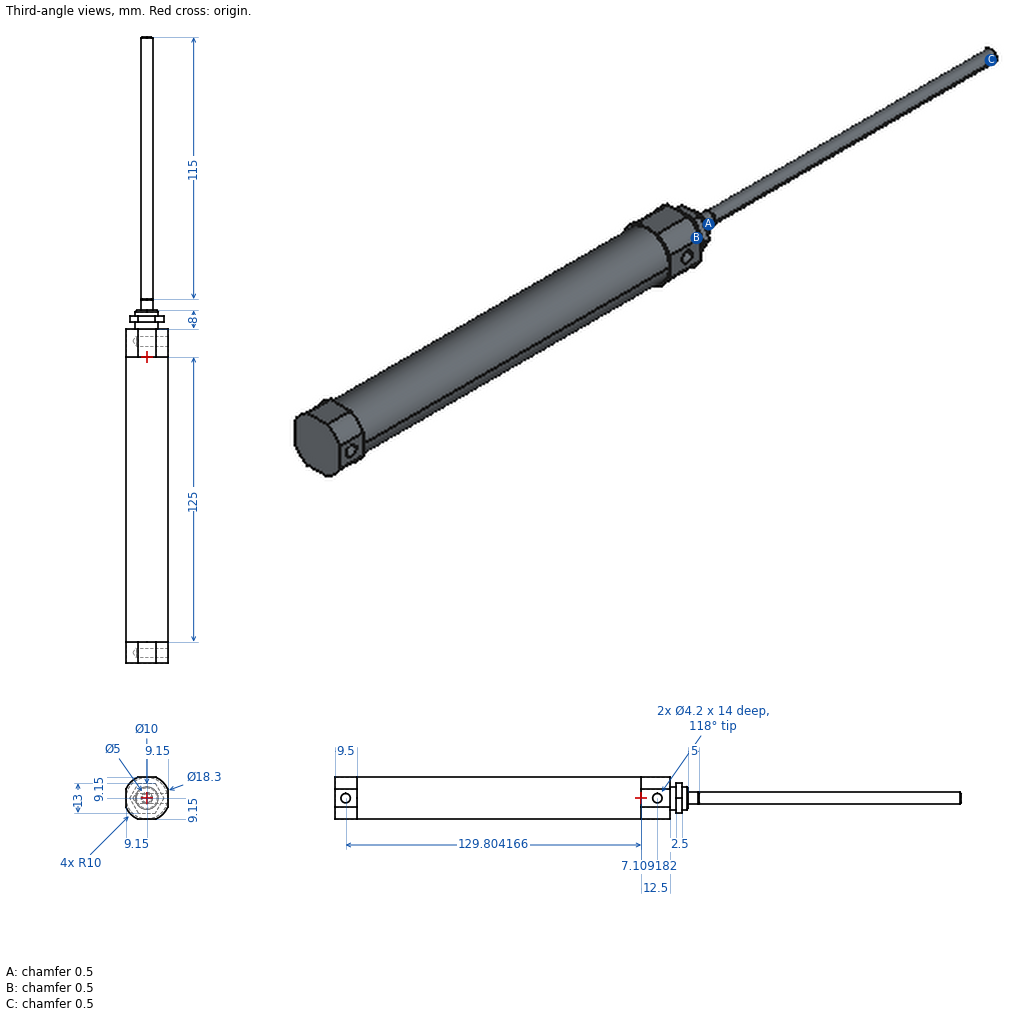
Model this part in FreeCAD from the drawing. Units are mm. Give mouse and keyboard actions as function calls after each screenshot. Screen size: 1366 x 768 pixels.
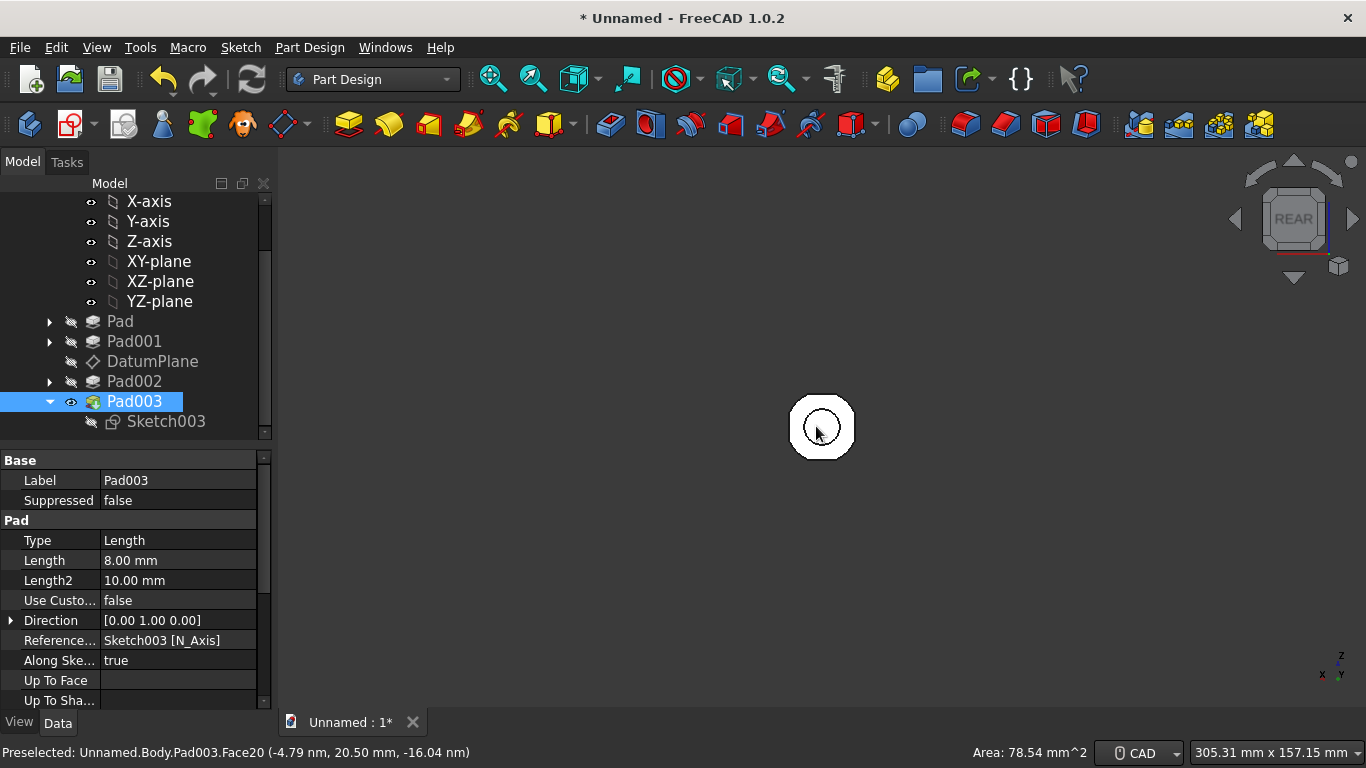
click(70, 124)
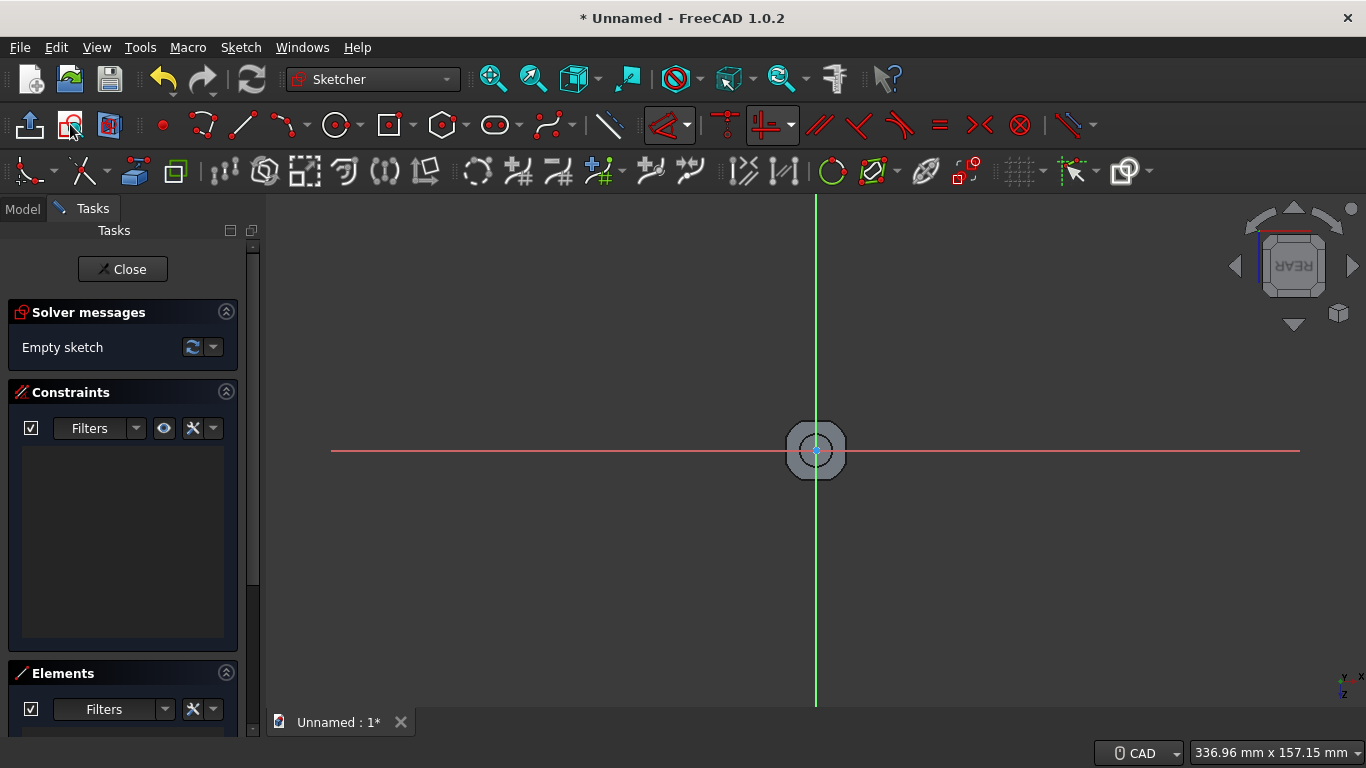
scroll(820, 451, up, 15)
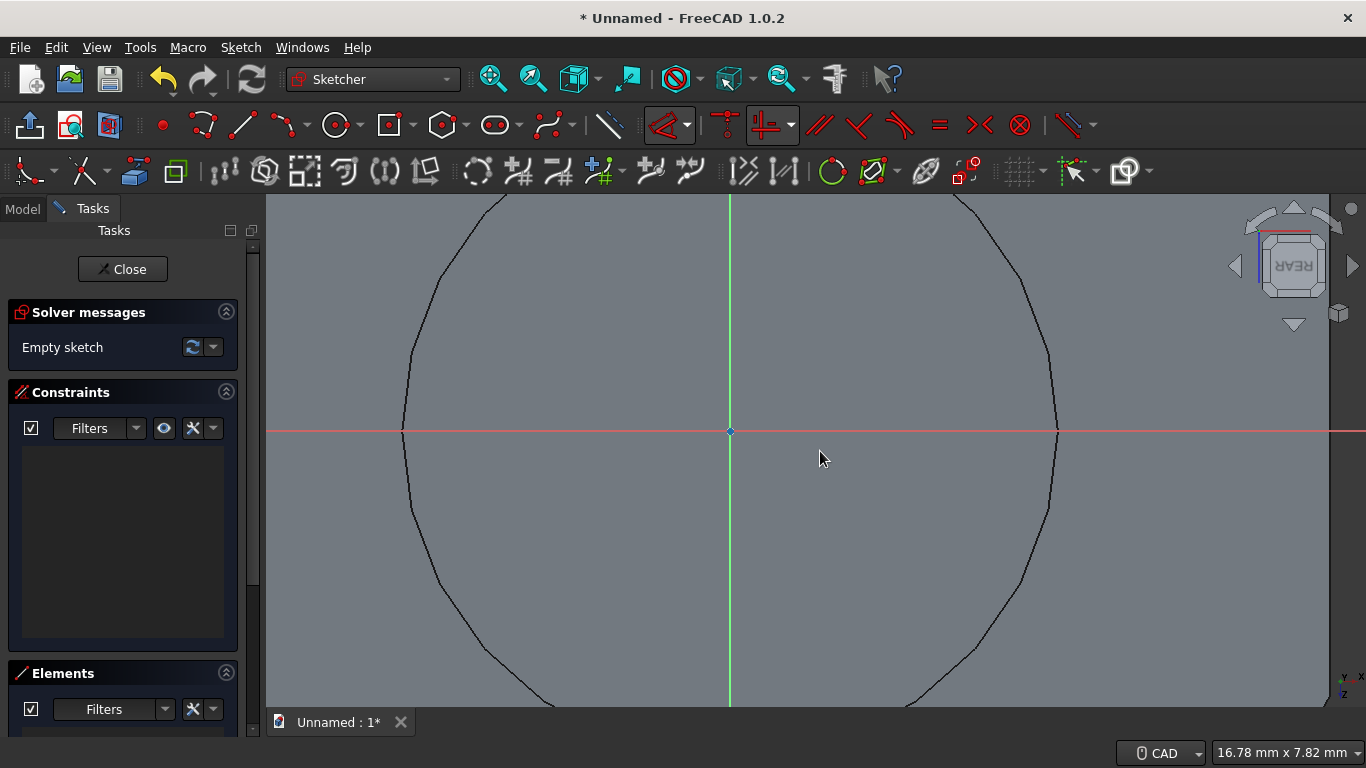
key(g)
key(c)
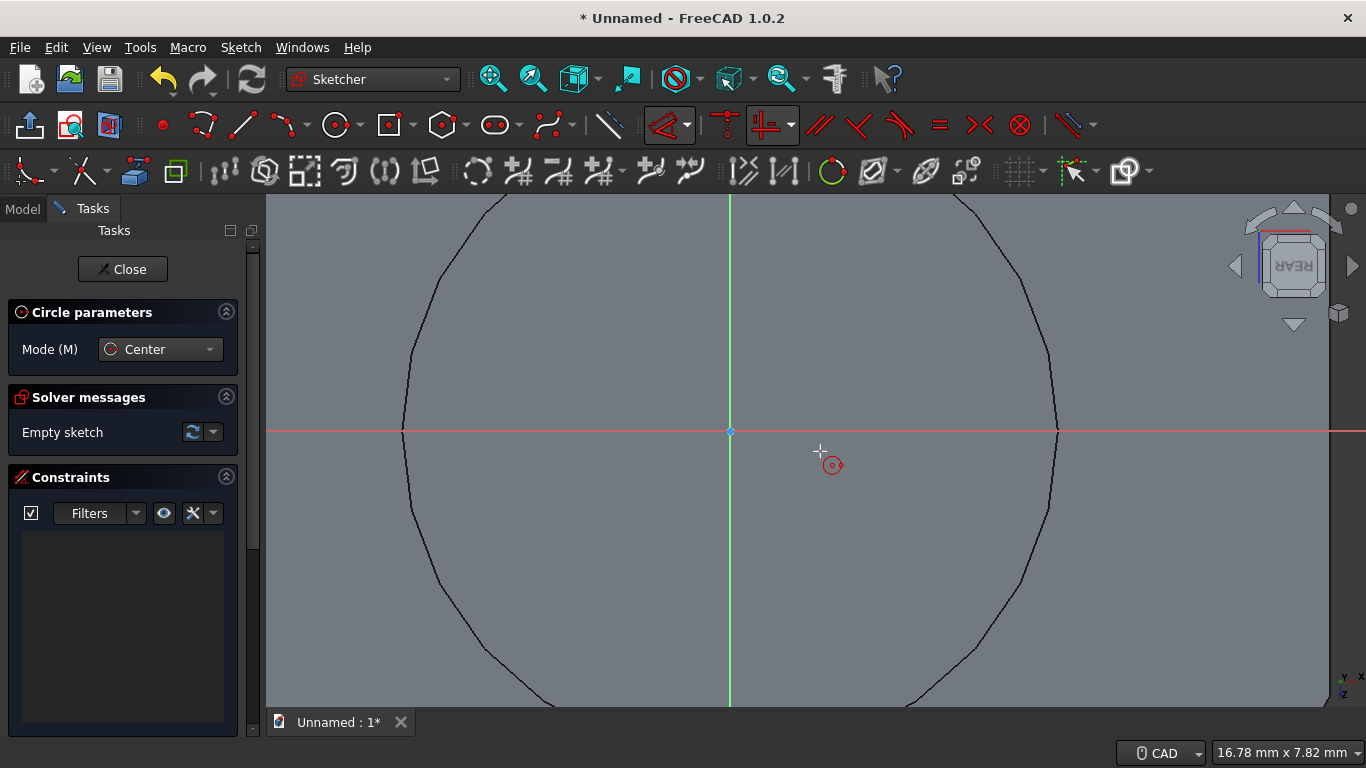
click(730, 431)
click(846, 315)
key(Escape)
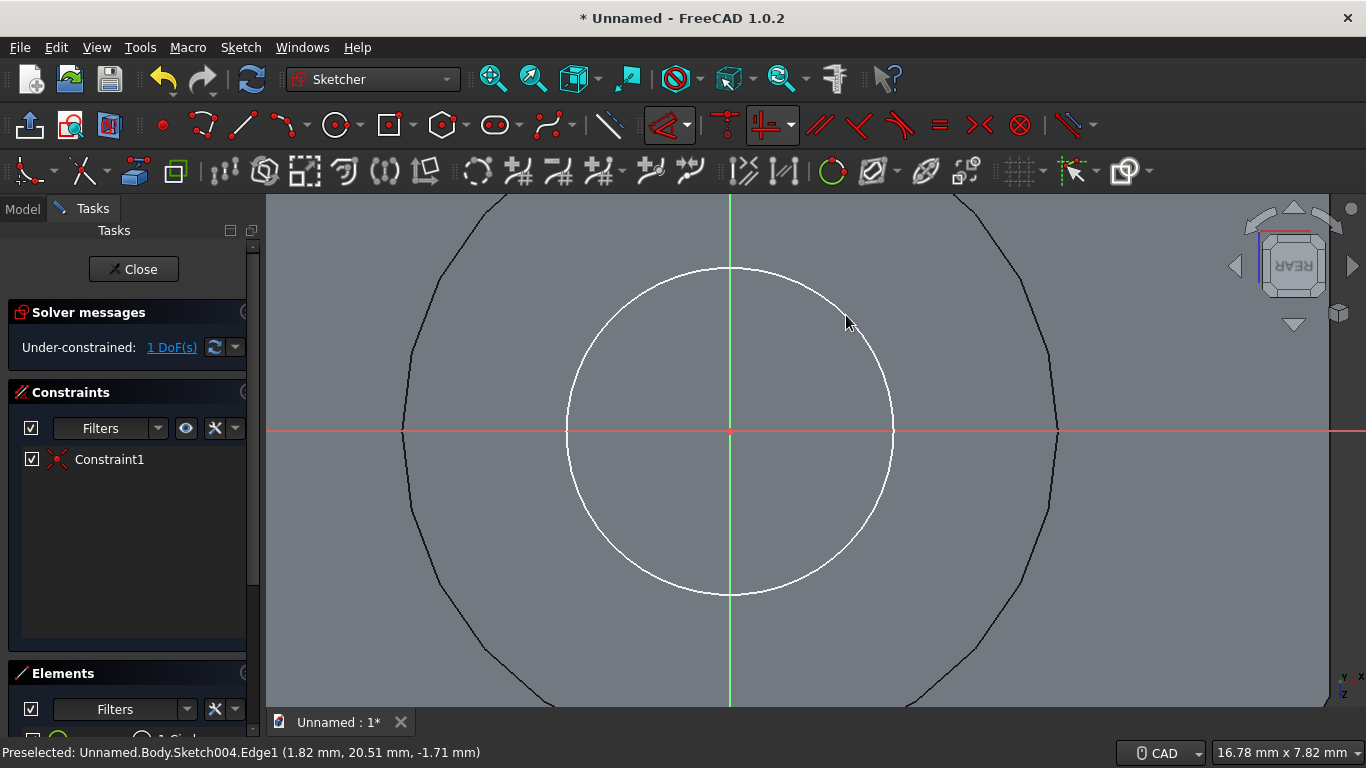
key(d)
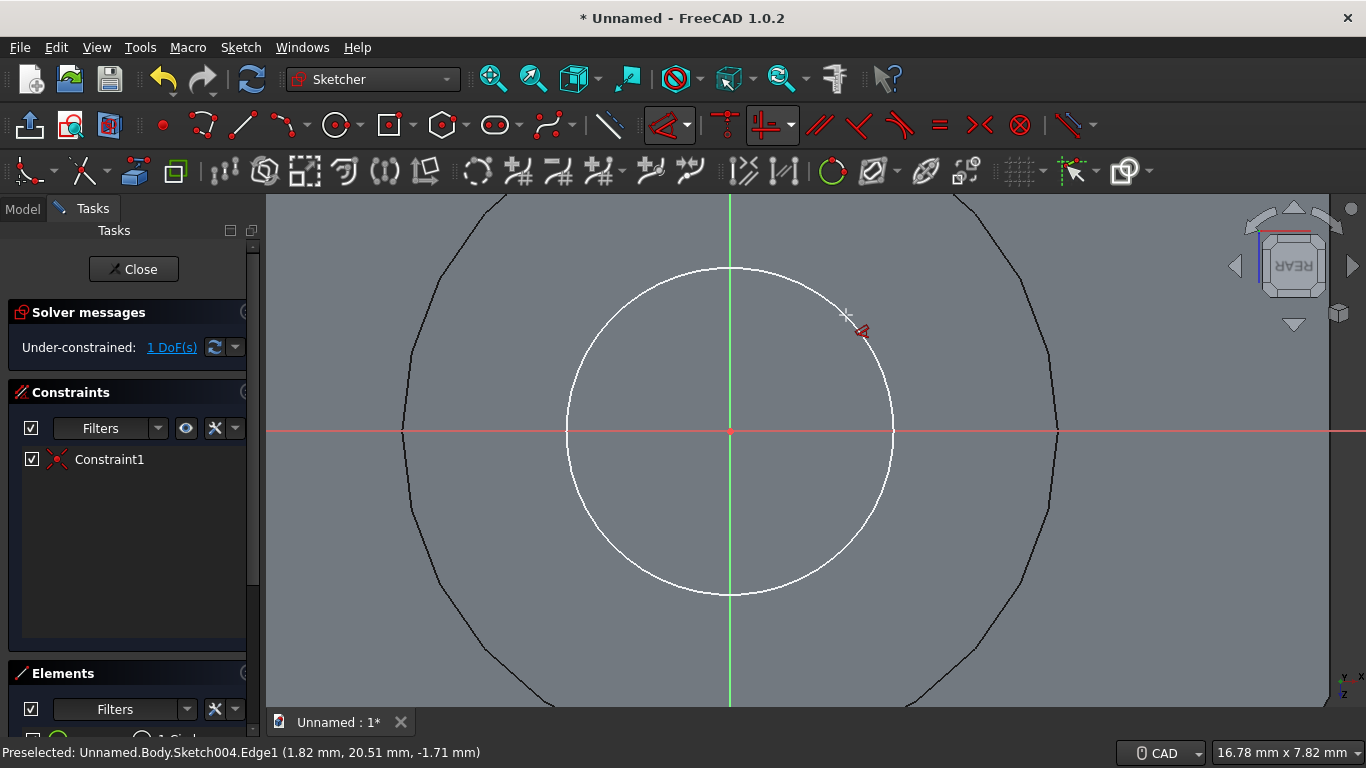
click(845, 315)
click(867, 292)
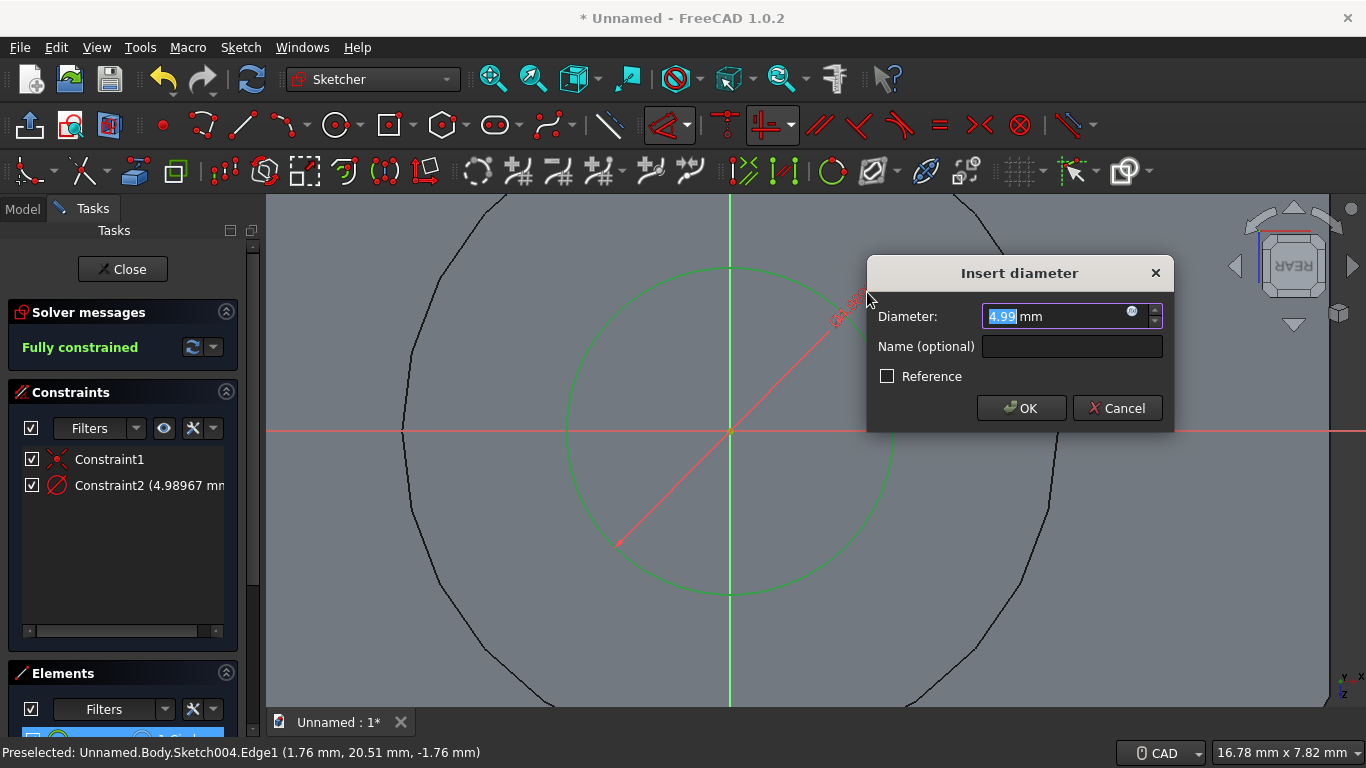
text(5)
key(Return)
key(Escape)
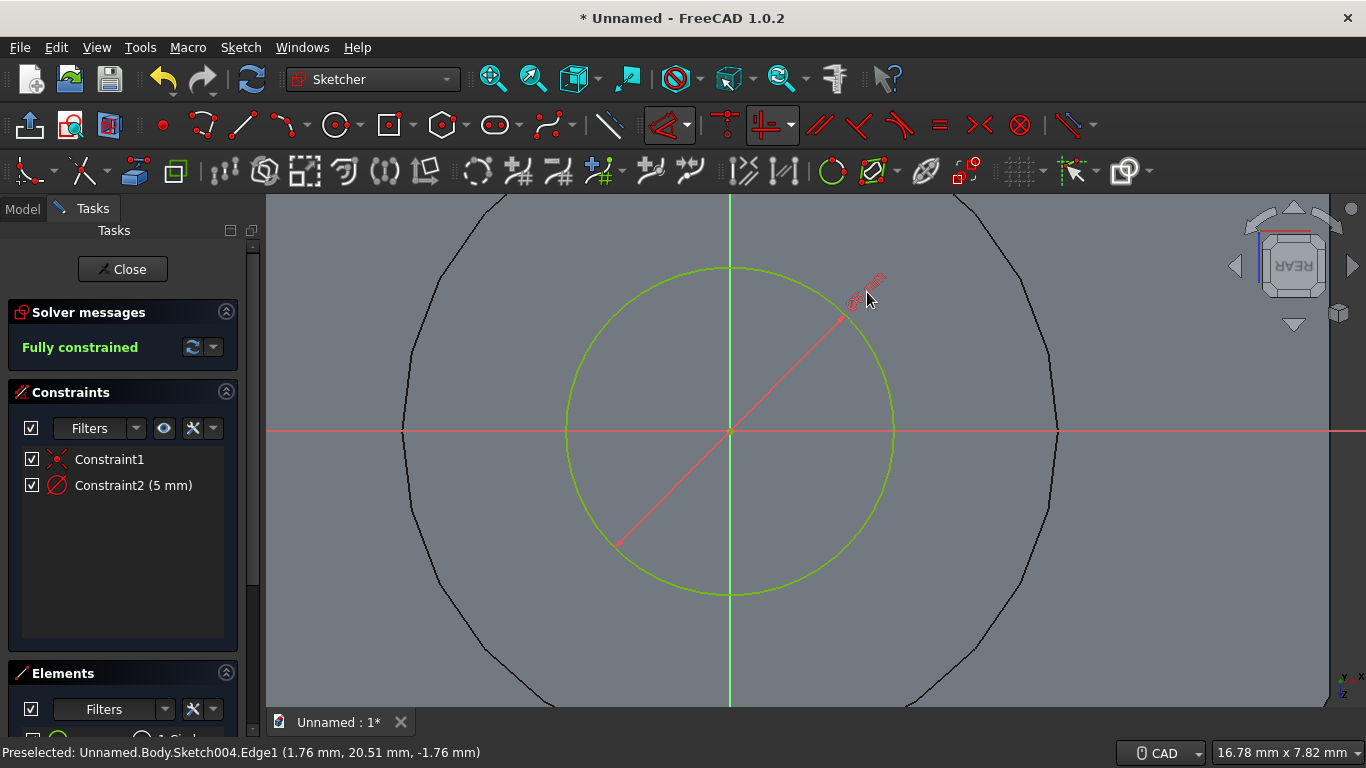
click(123, 269)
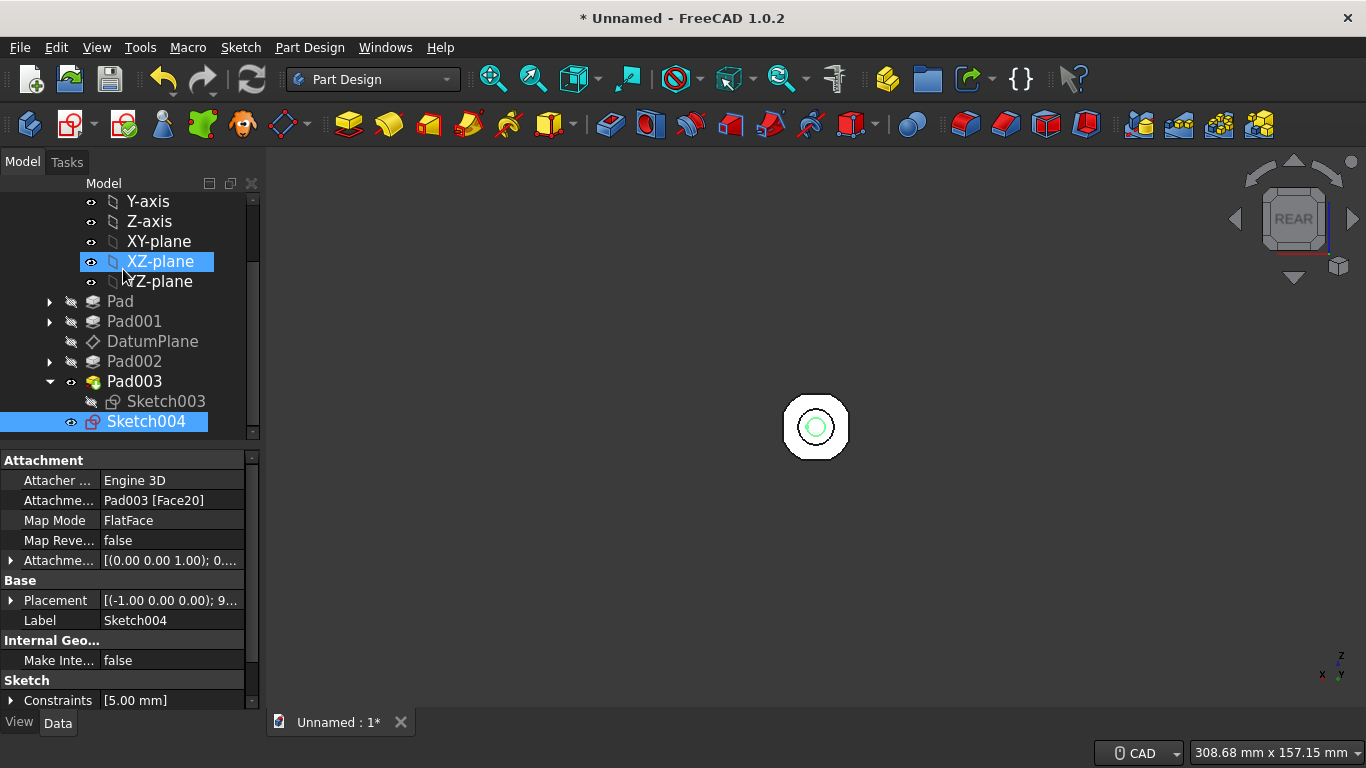
click(350, 124)